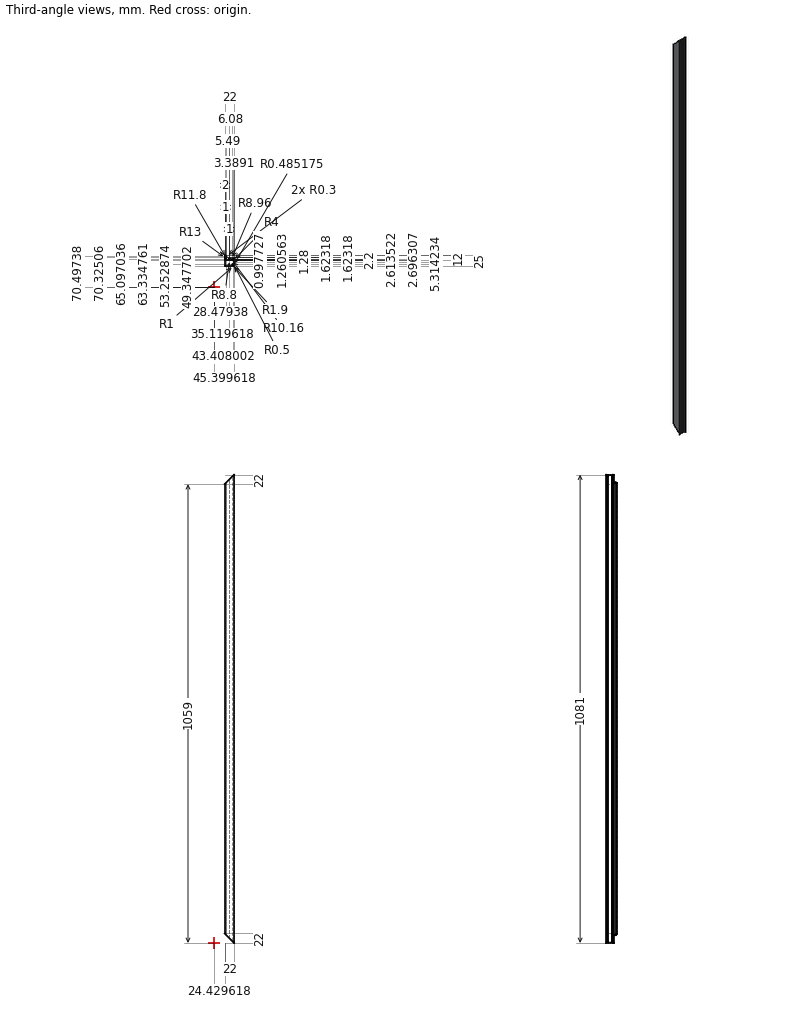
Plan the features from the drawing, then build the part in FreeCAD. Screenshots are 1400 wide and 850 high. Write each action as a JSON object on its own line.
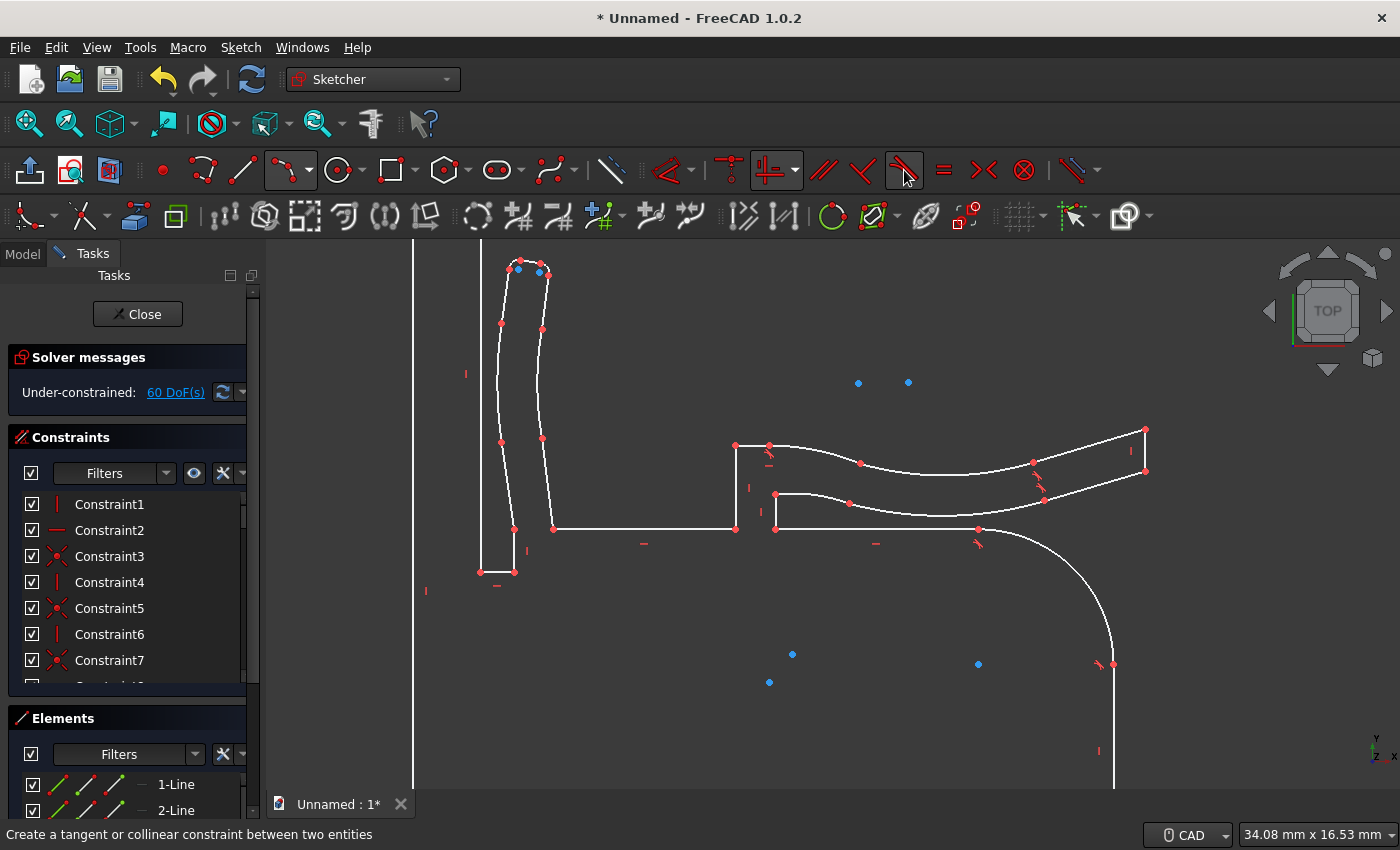
{"action": "left_click", "coordinate": [550, 502]}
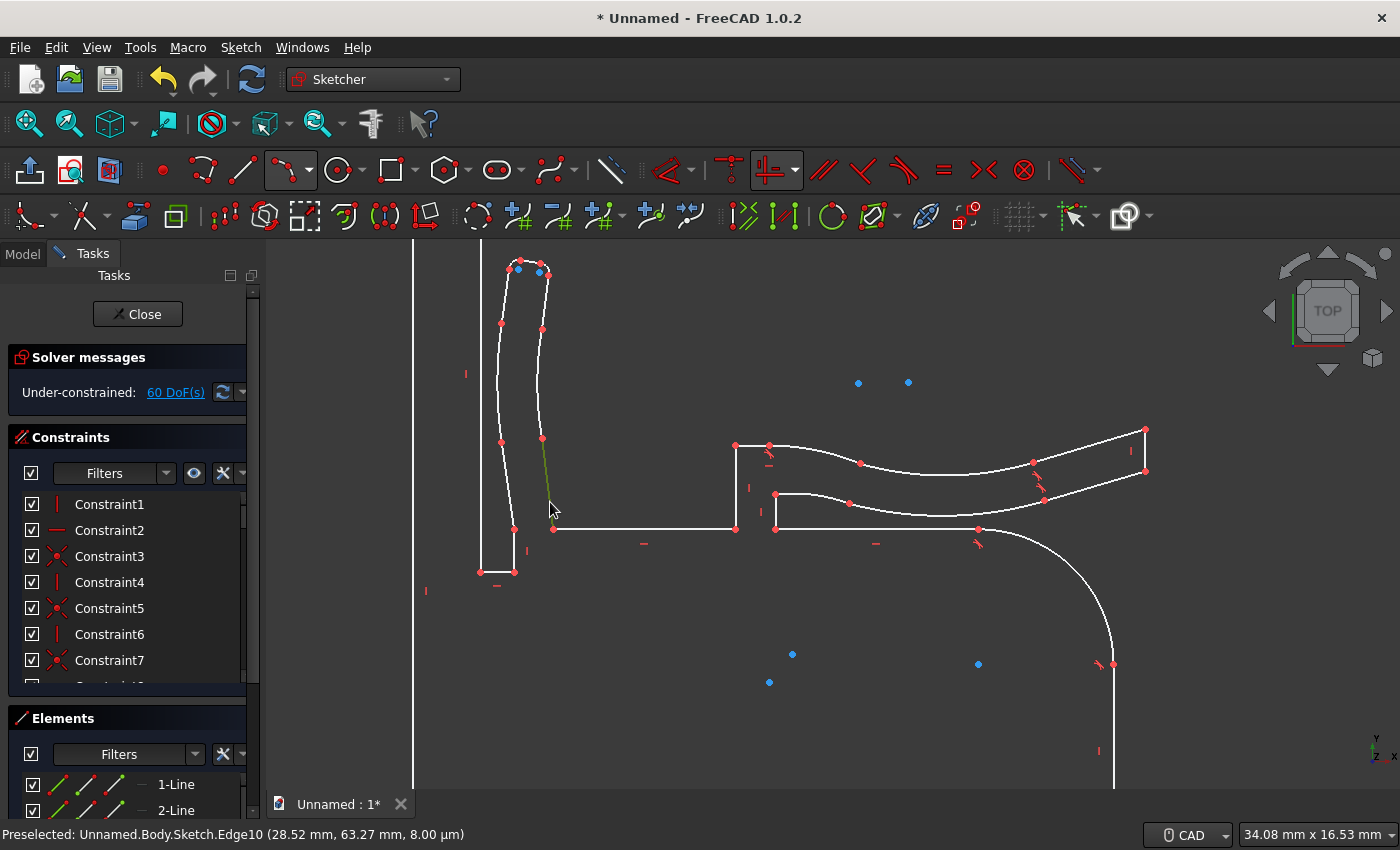
{"action": "left_click", "coordinate": [538, 362]}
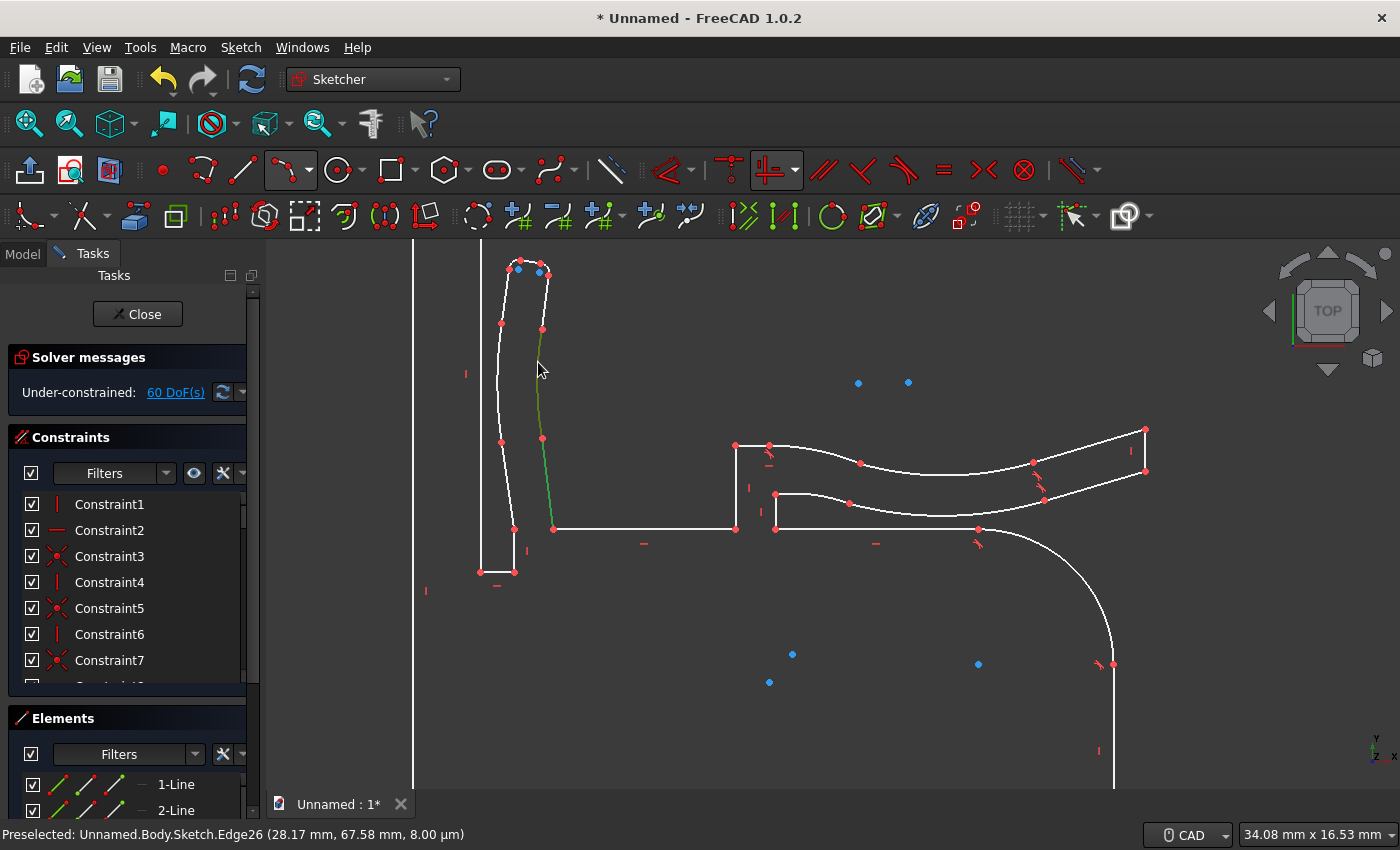
{"action": "left_click", "coordinate": [904, 170]}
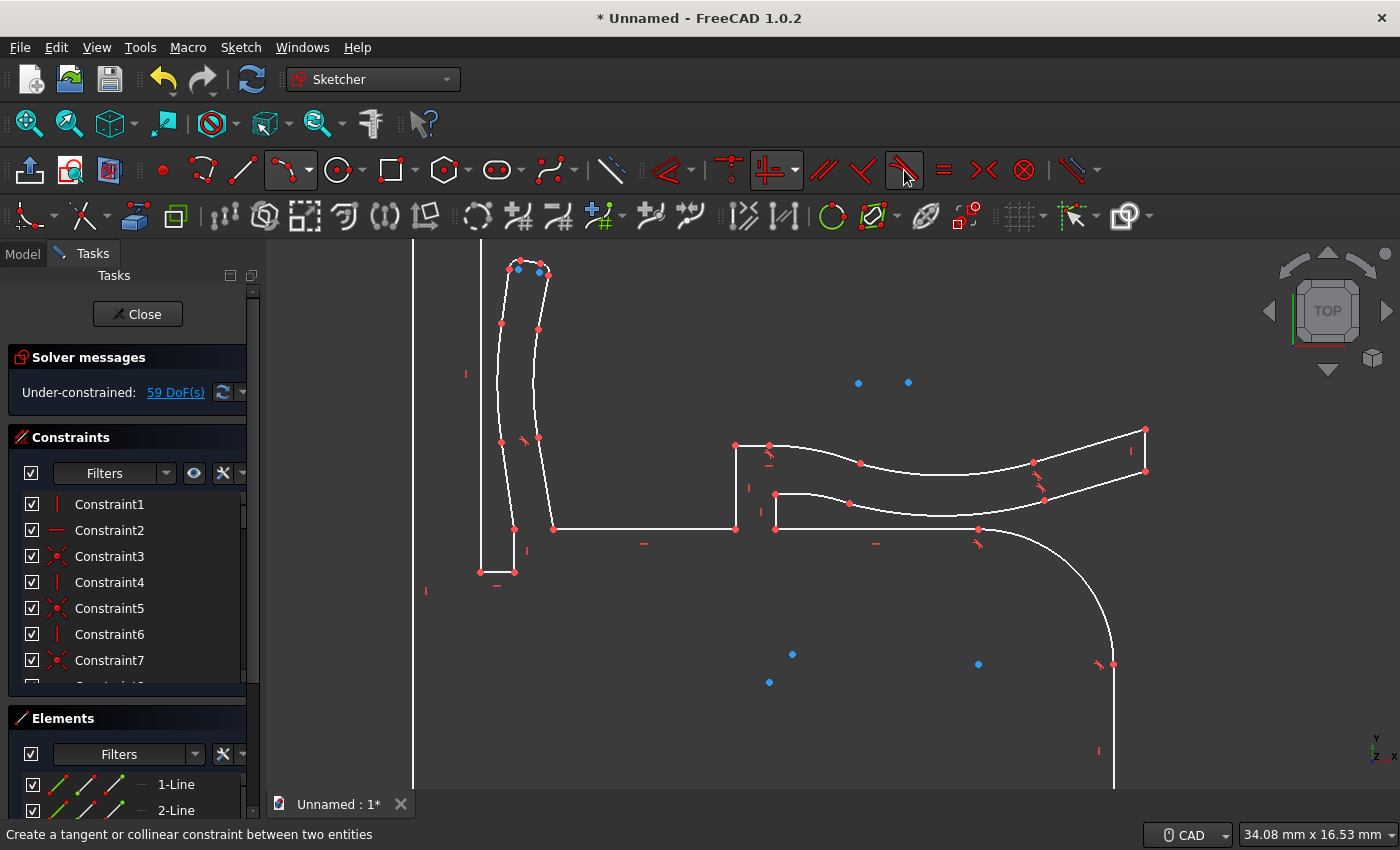
{"action": "left_click", "coordinate": [541, 313]}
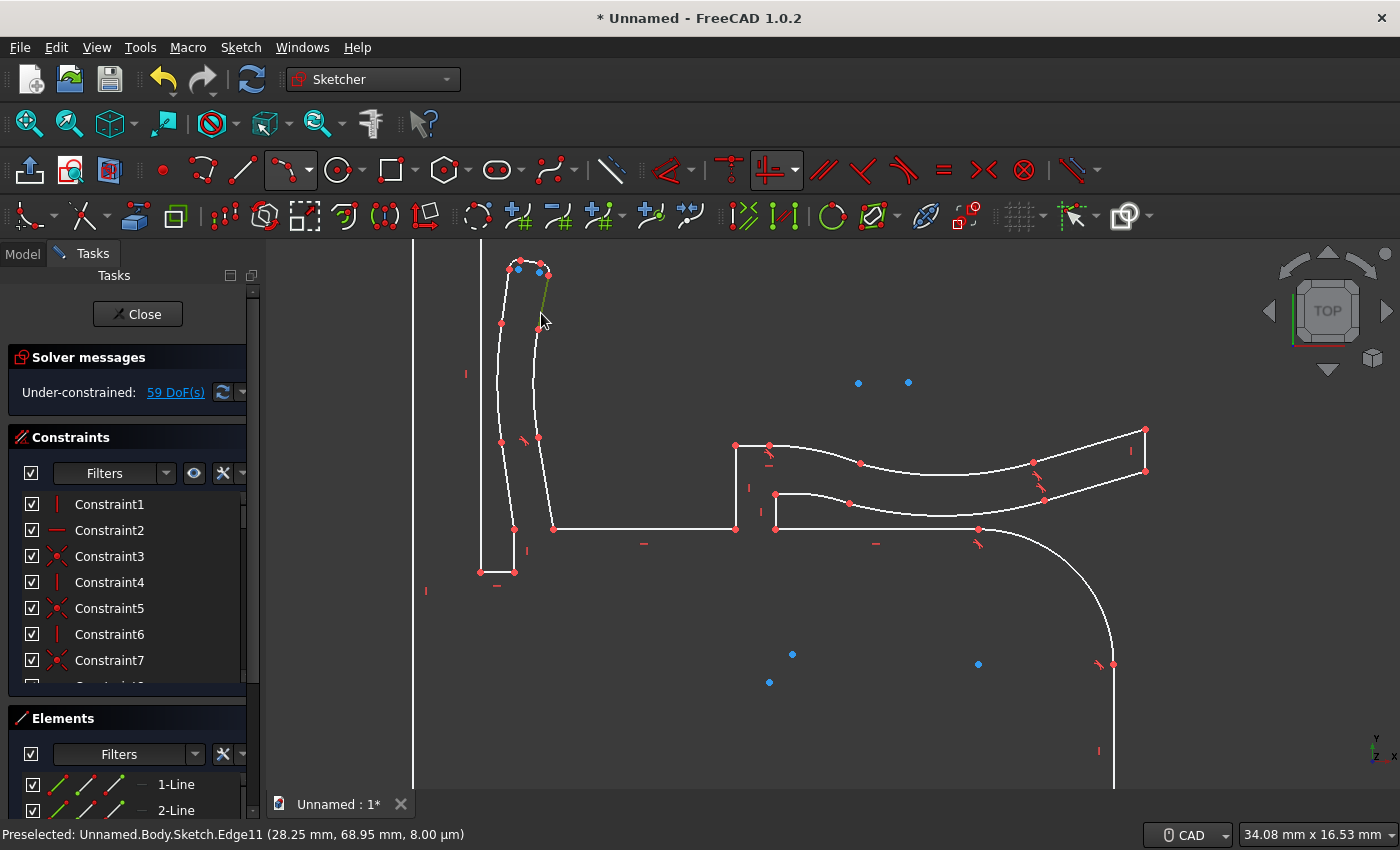
{"action": "left_click", "coordinate": [534, 362]}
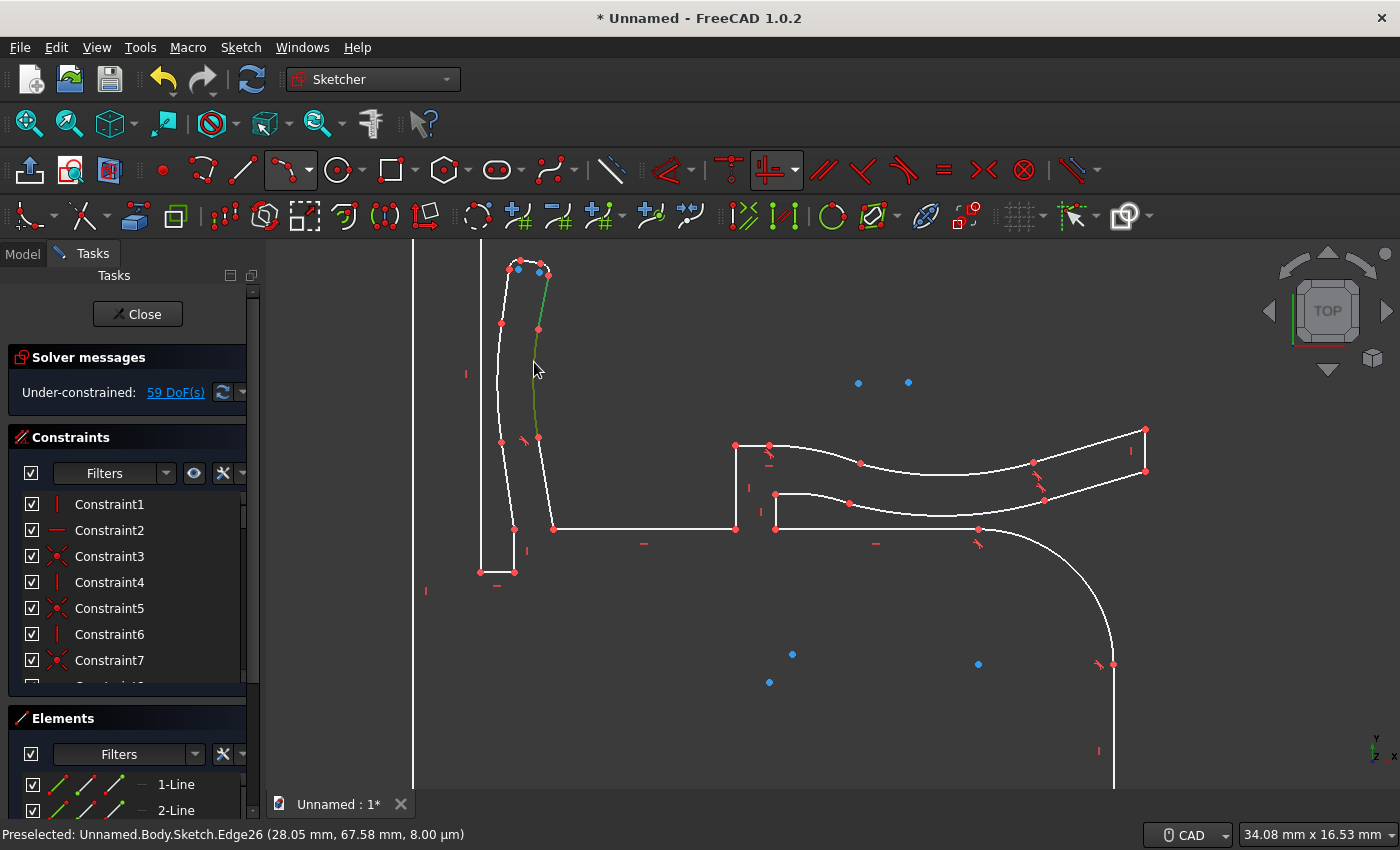
{"action": "left_click", "coordinate": [904, 170]}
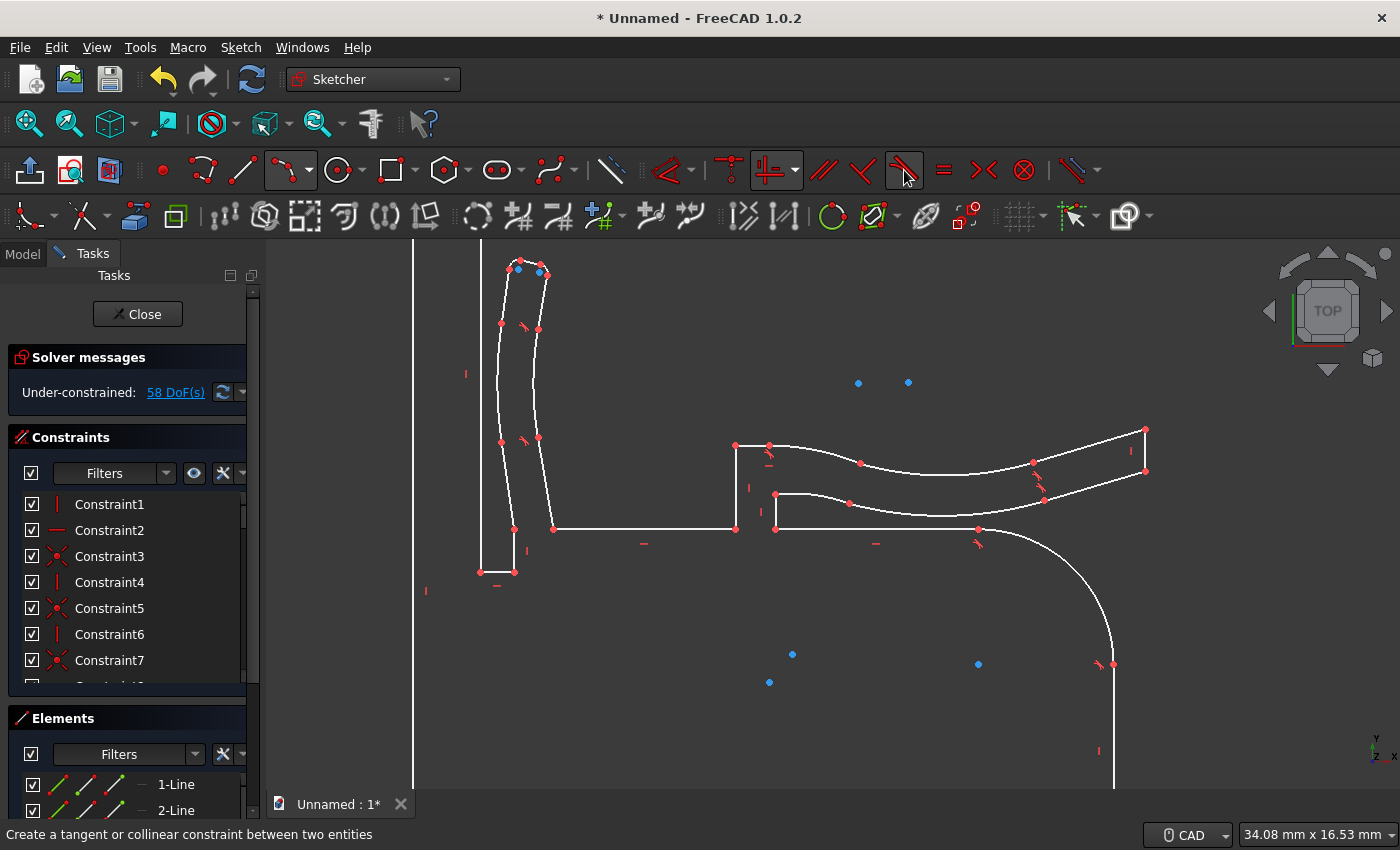
{"action": "left_click", "coordinate": [541, 313]}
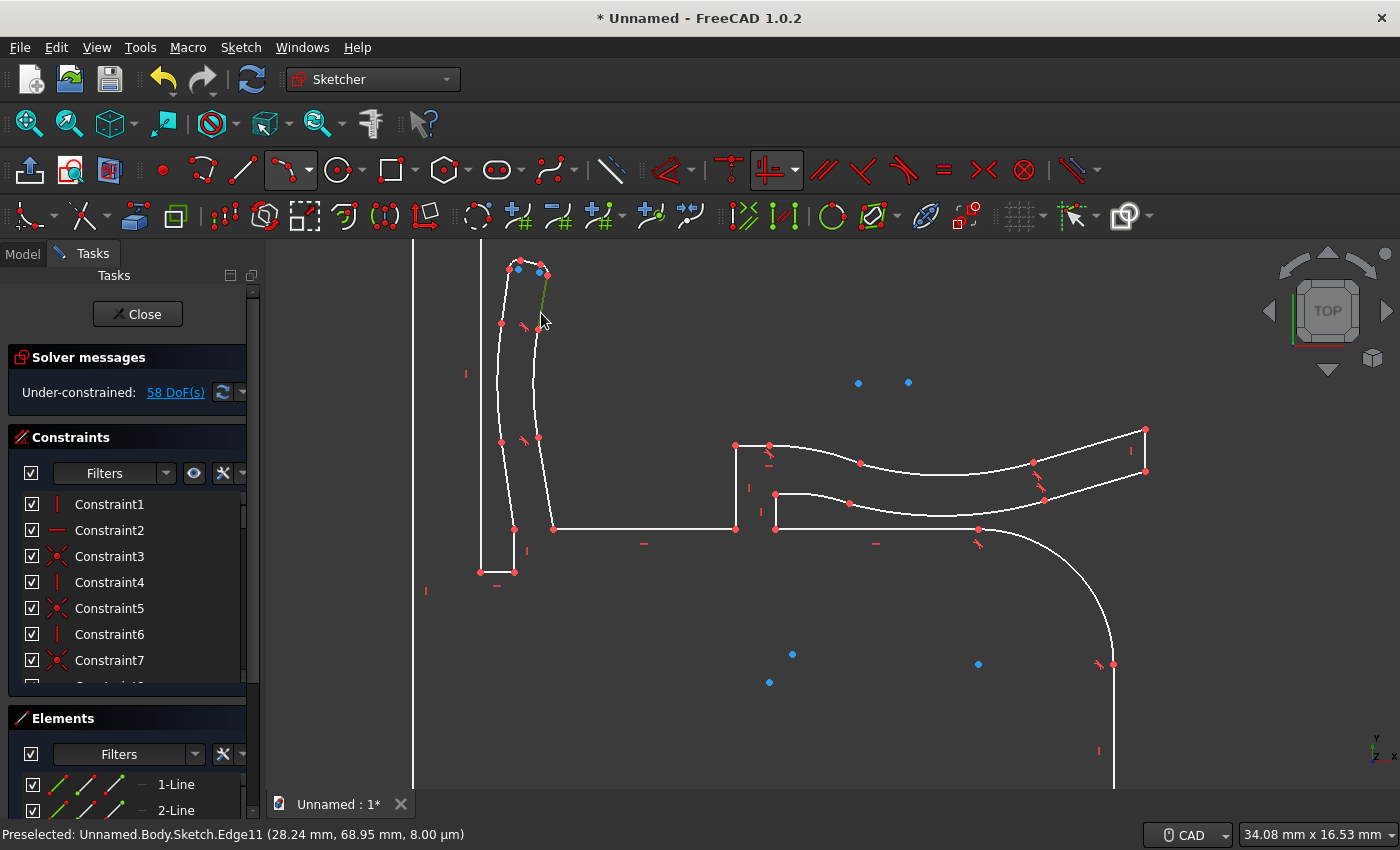
{"action": "scroll", "coordinate": [546, 268], "scroll_direction": "up", "scroll_amount": 4}